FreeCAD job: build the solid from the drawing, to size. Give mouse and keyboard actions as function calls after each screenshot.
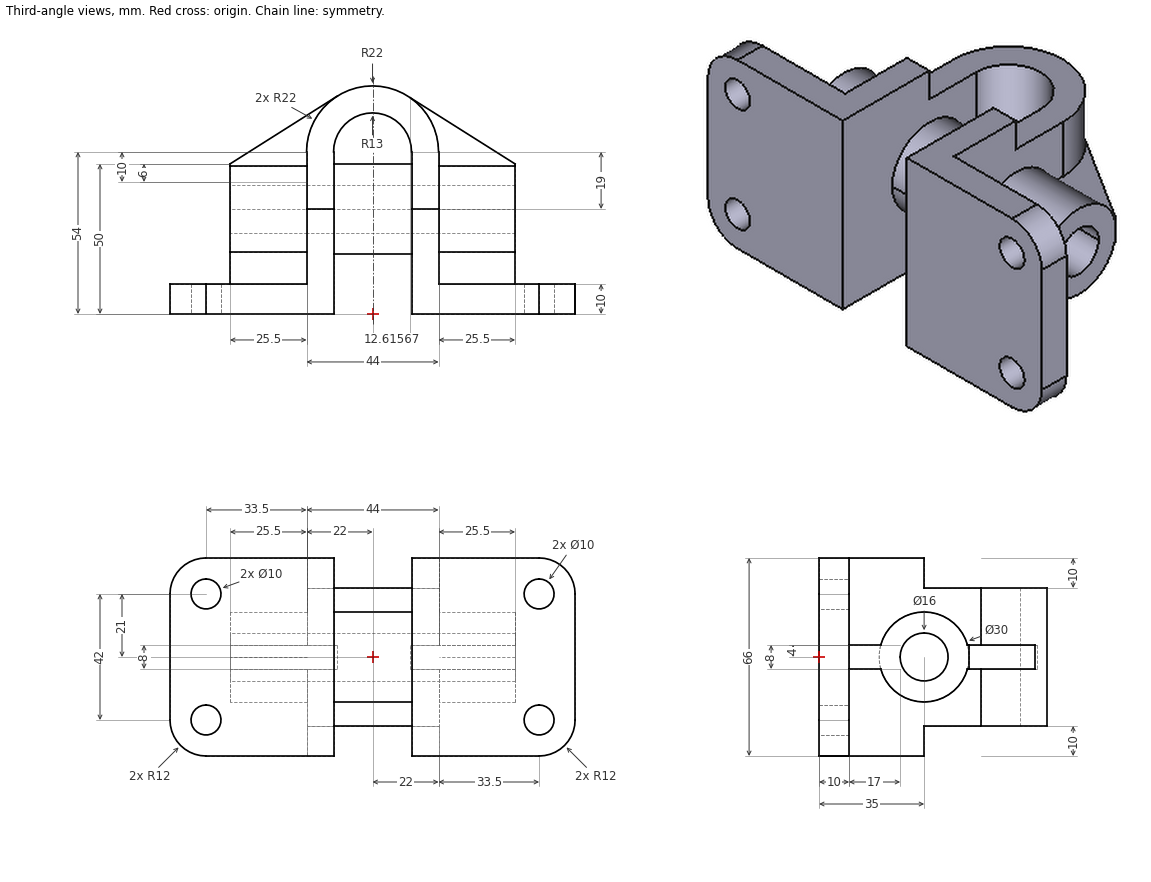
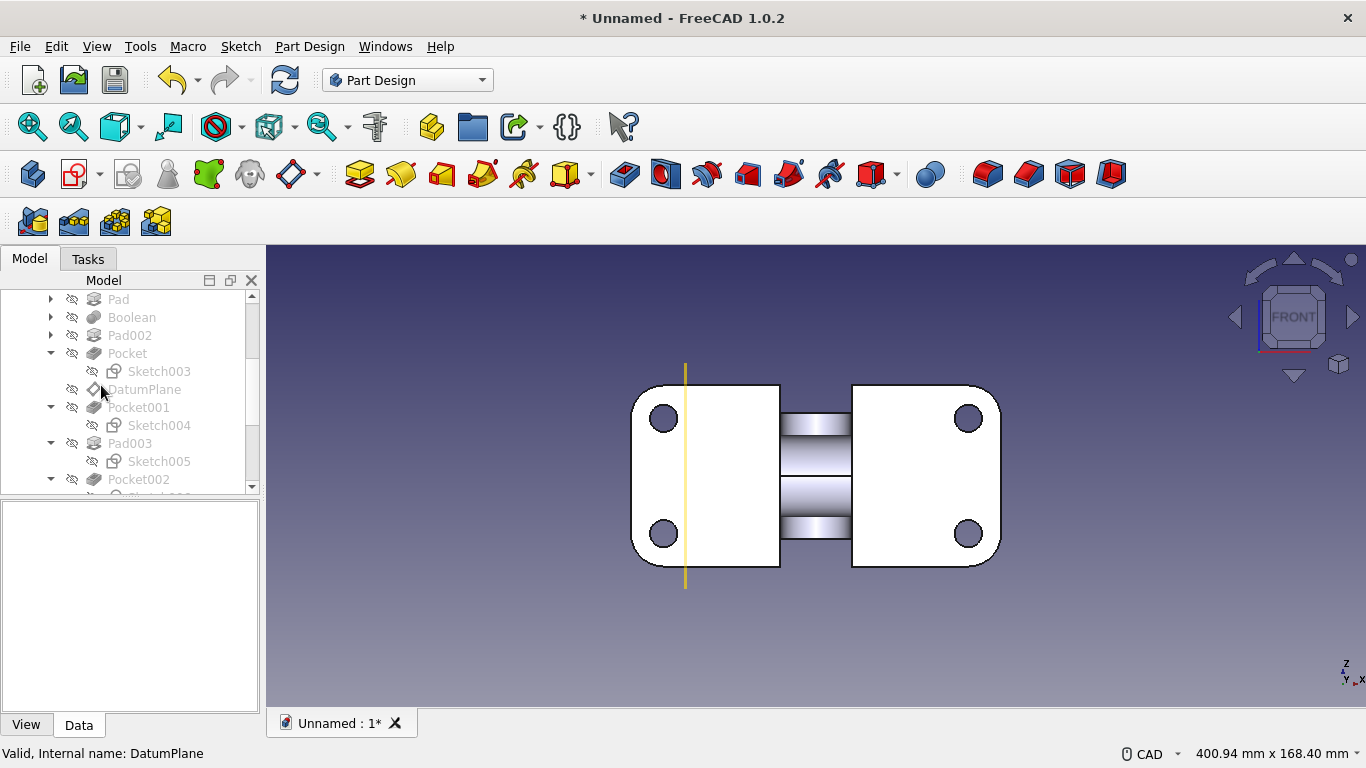
scroll(141, 385, up, 15)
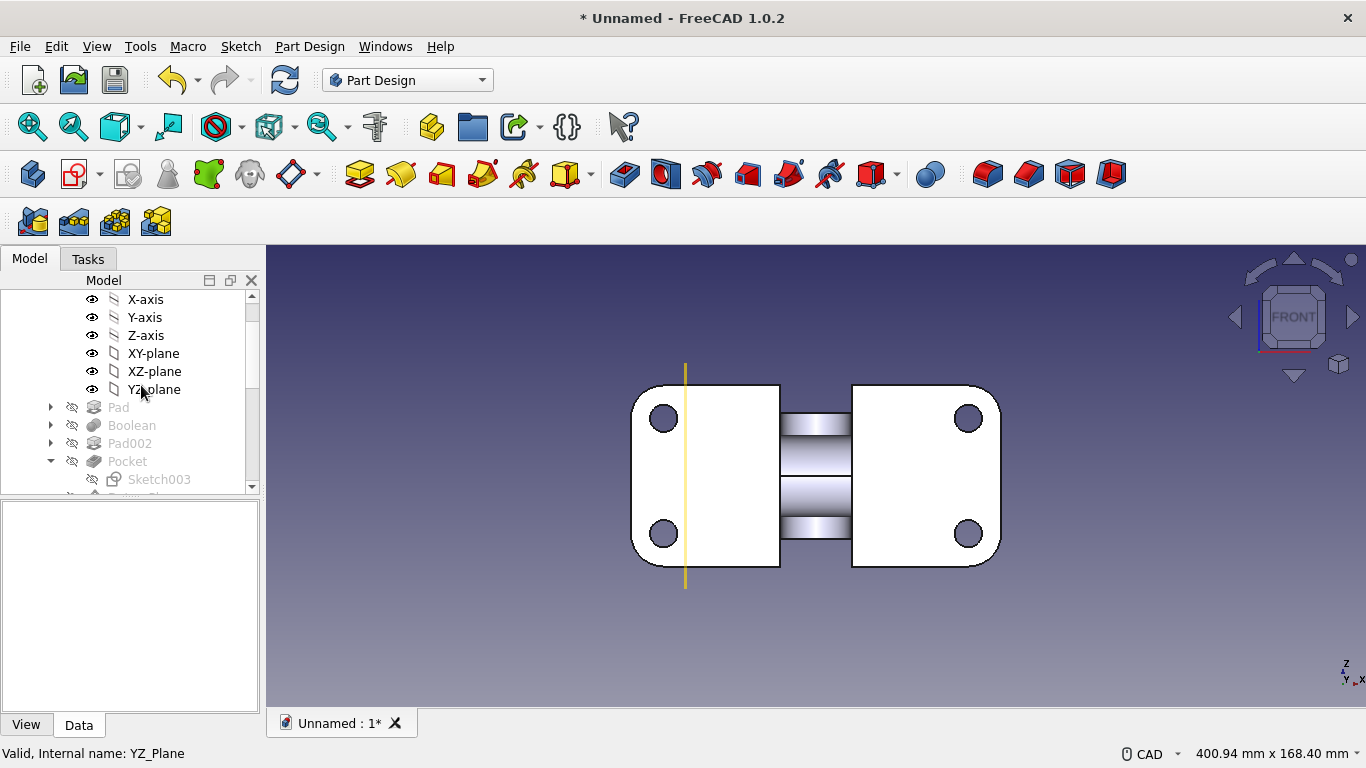
scroll(101, 385, down, 6)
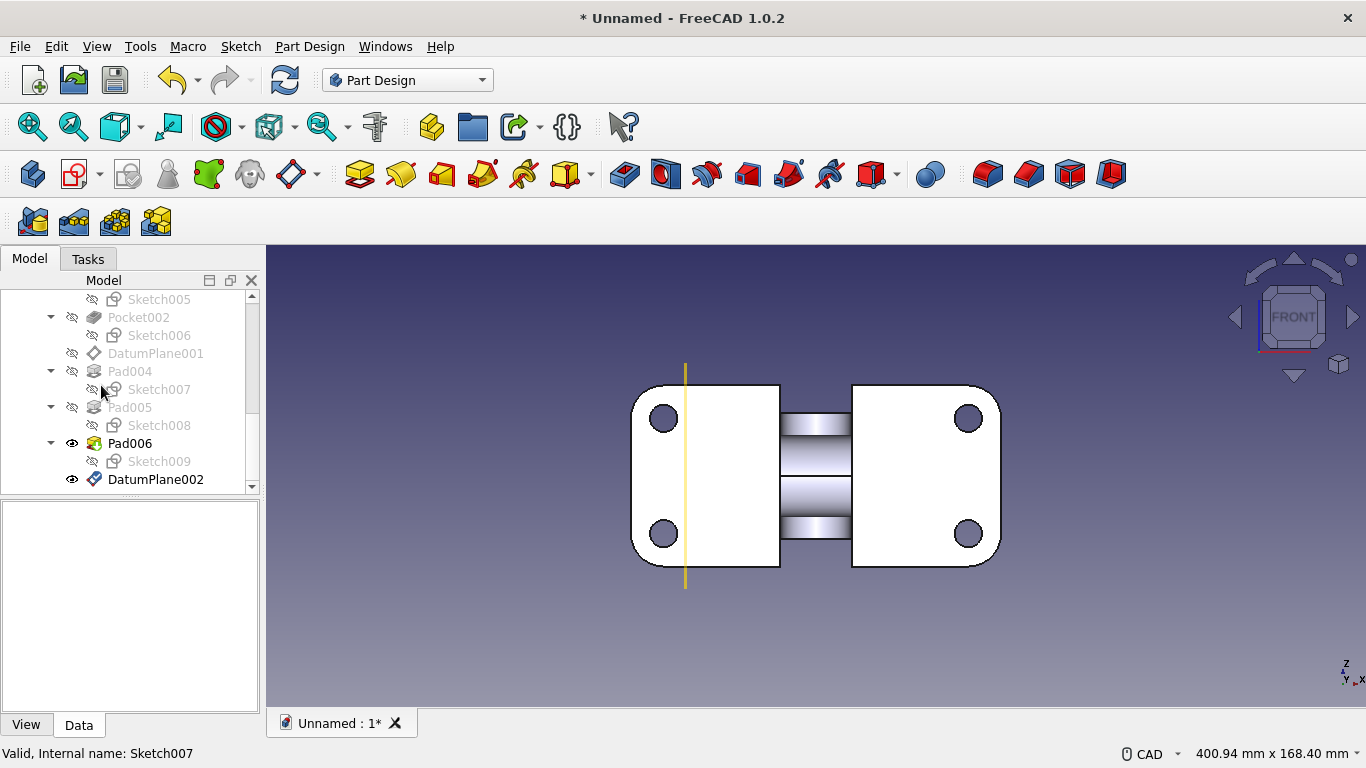
click(117, 479)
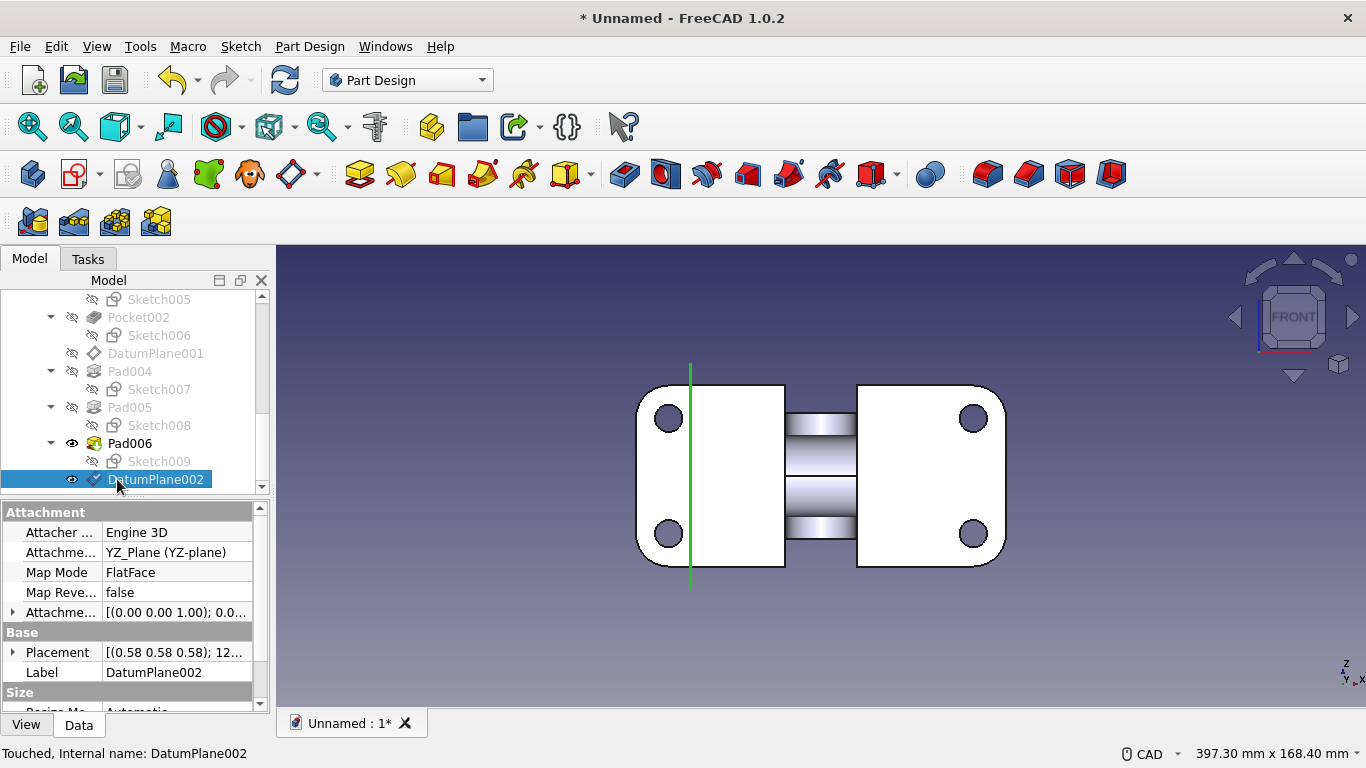
click(74, 174)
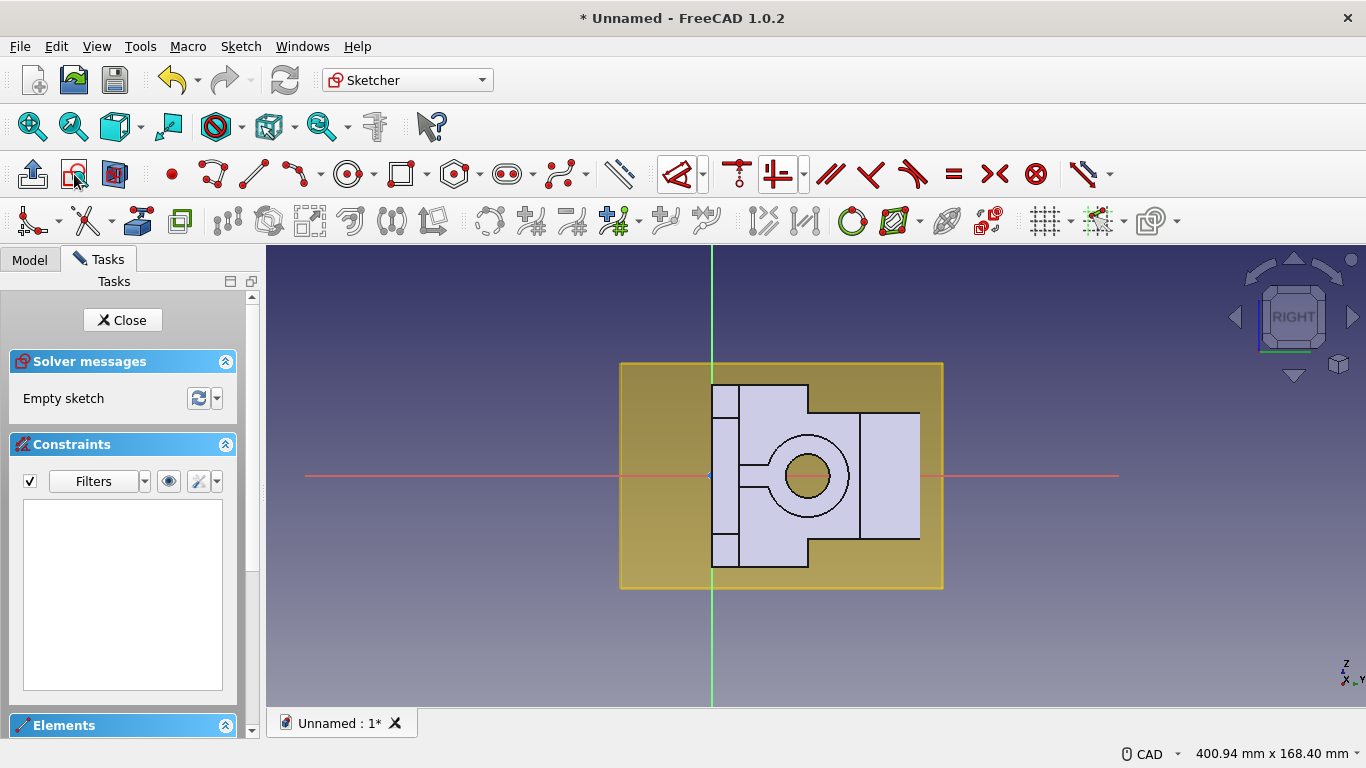
click(115, 174)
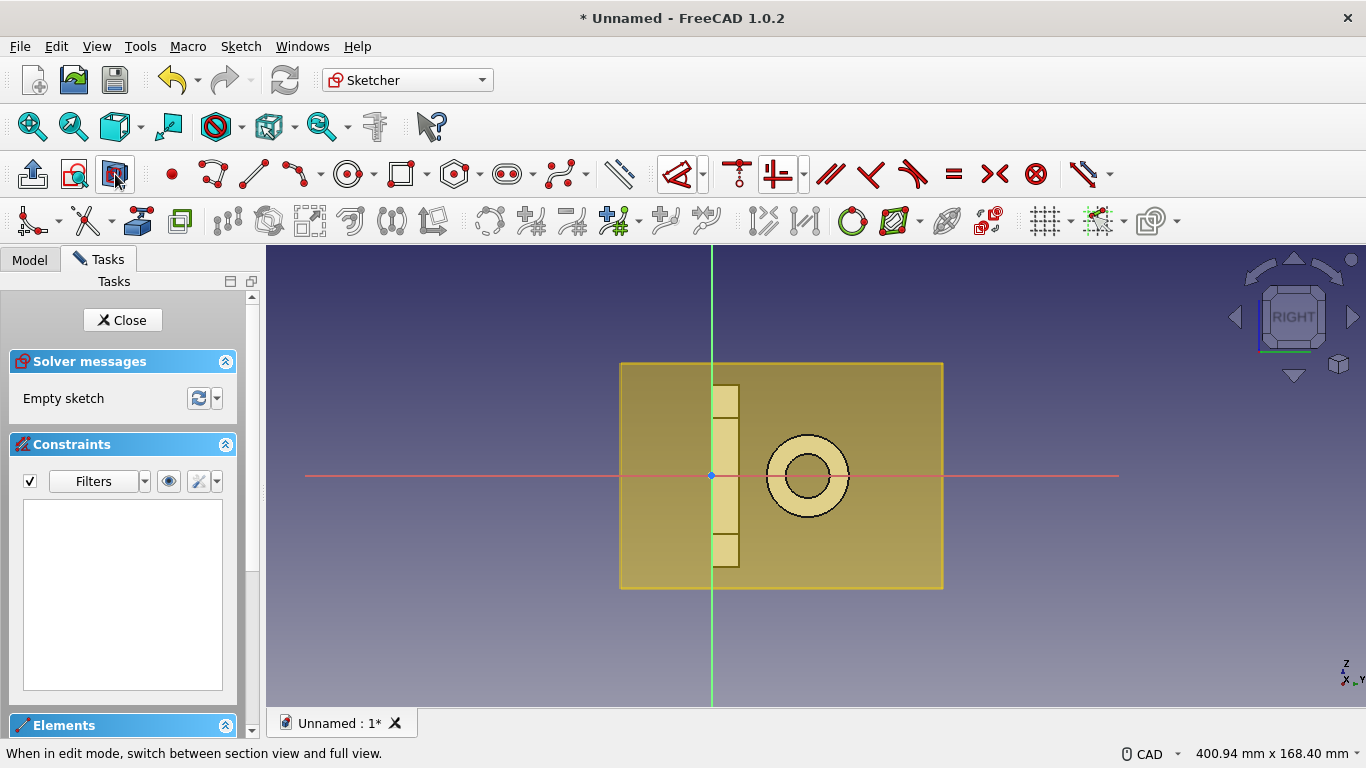
scroll(749, 476, up, 11)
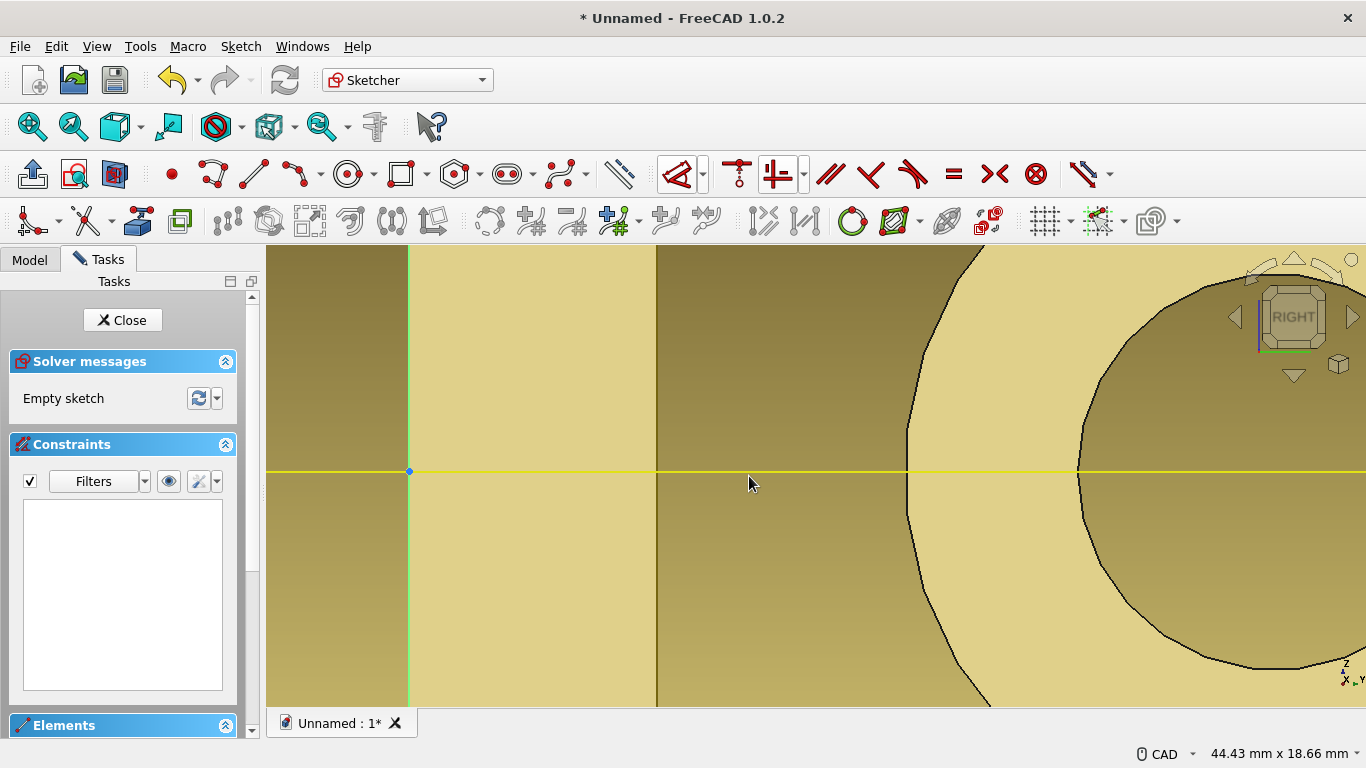
click(400, 174)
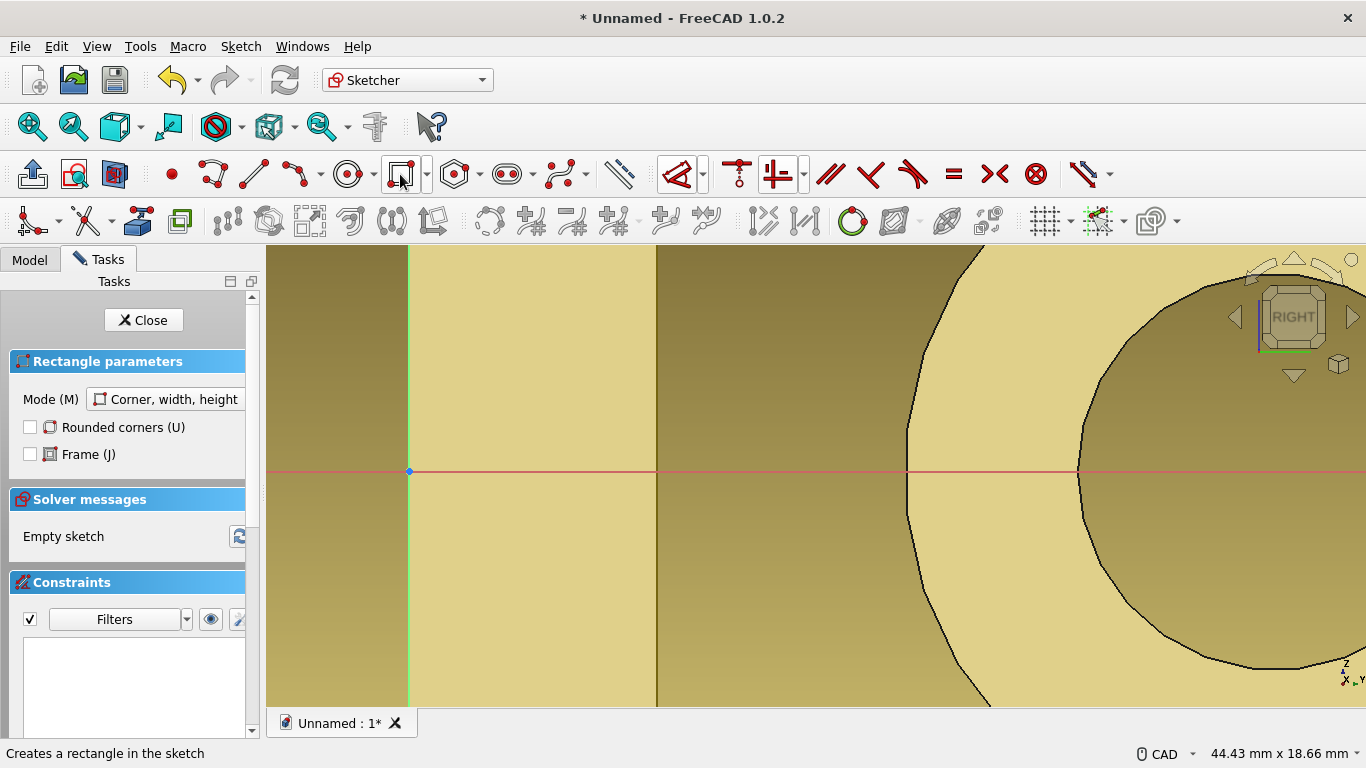
click(657, 373)
move(1078, 571)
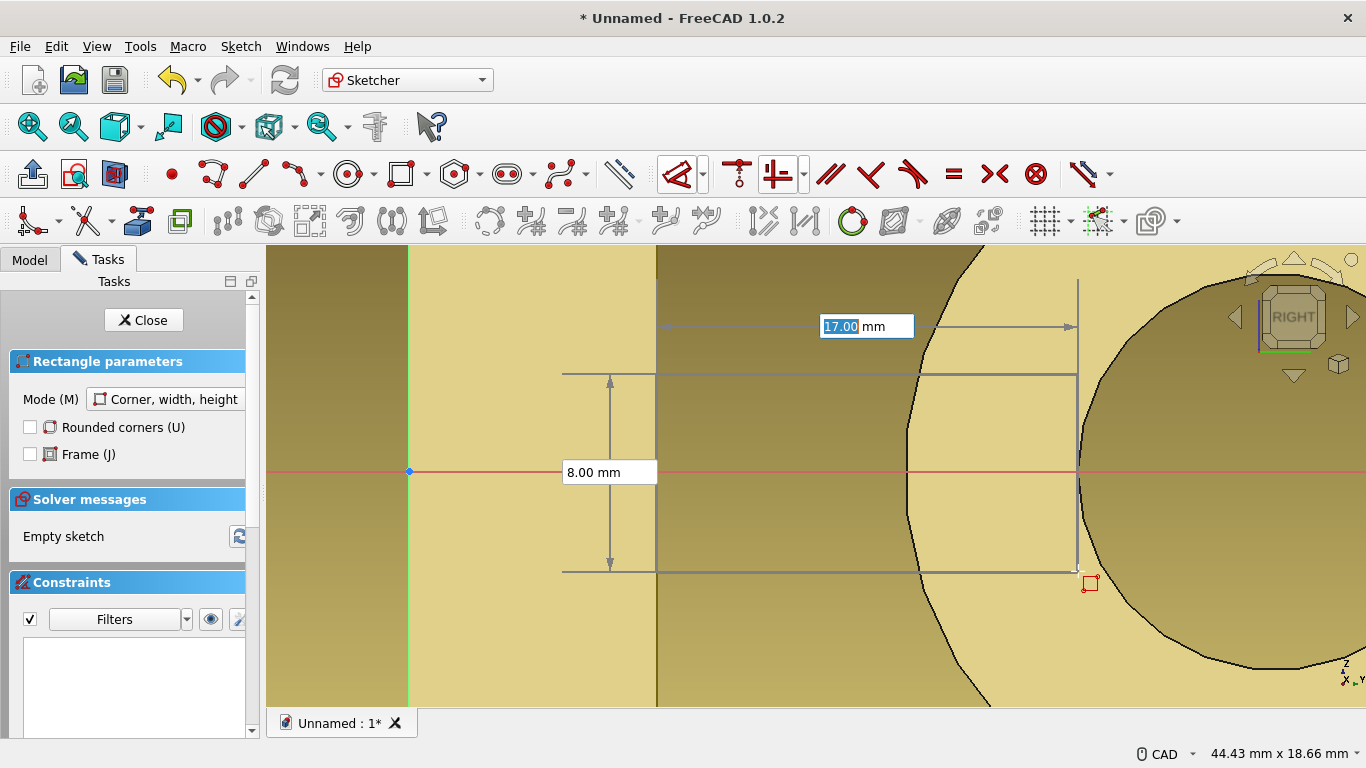
text(17)
key(Tab)
text(8)
key(Return)
key(Escape)